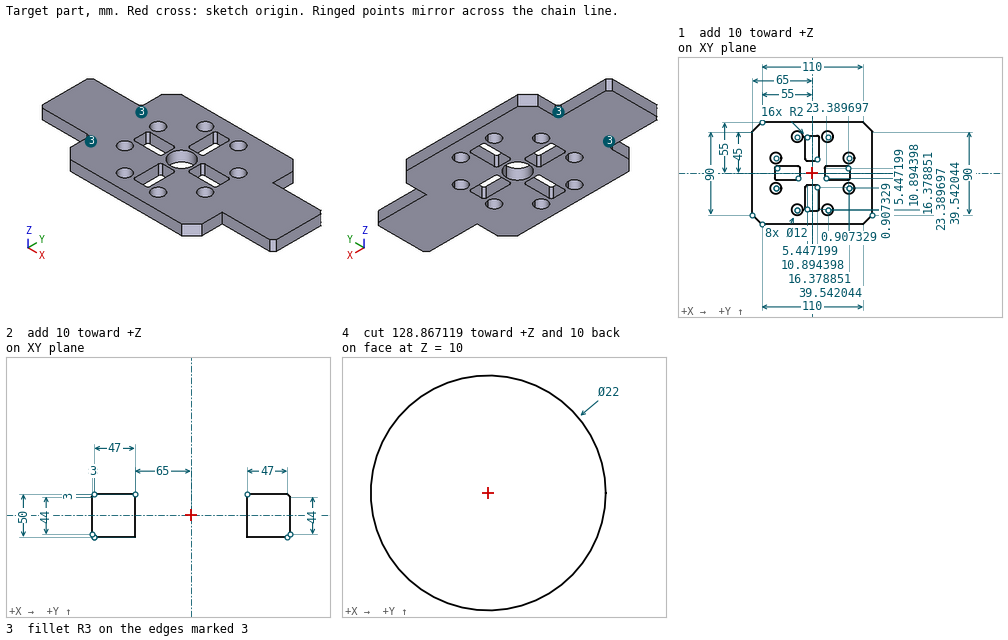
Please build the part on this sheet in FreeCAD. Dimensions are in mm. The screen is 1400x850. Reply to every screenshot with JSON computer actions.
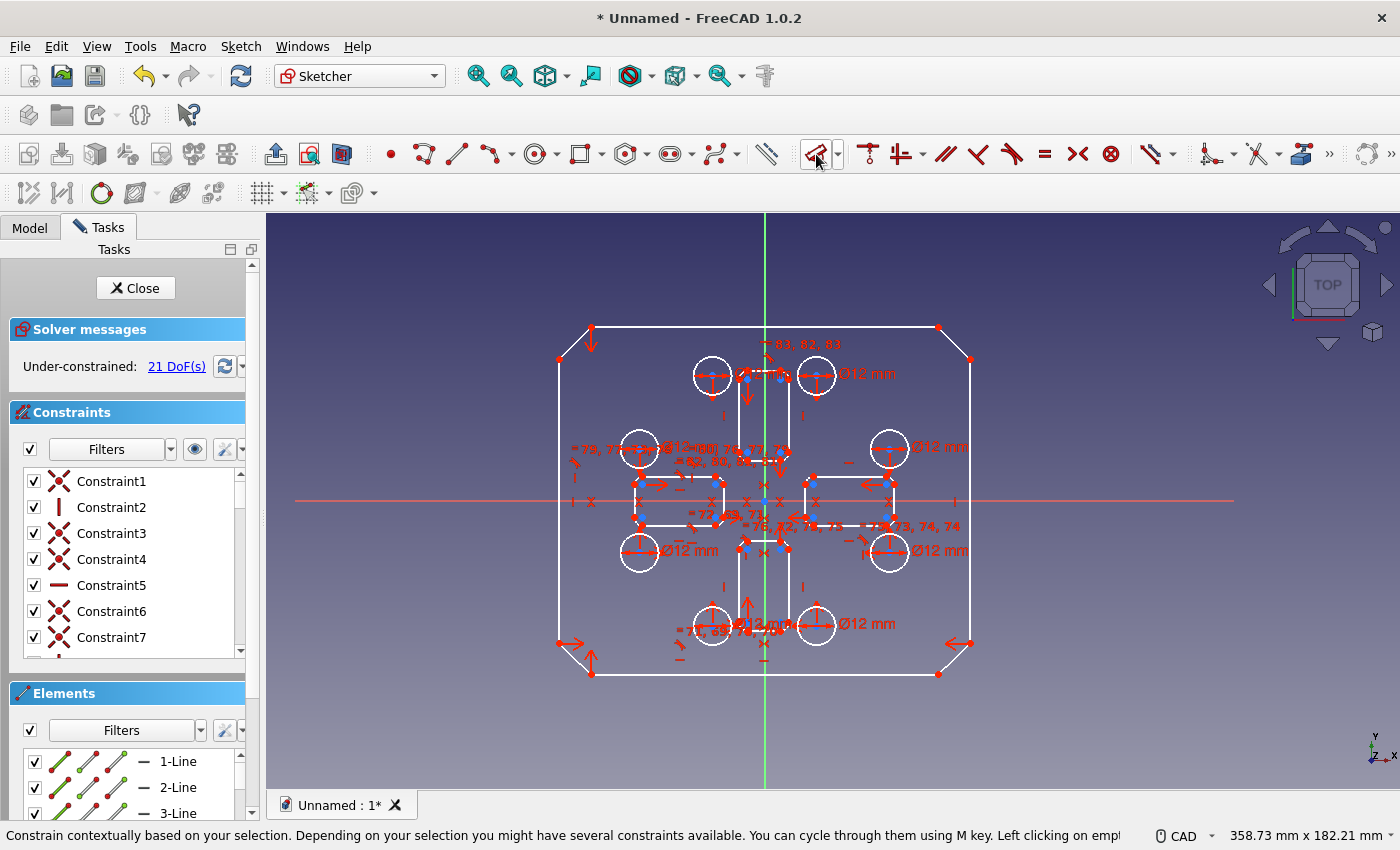
{"action": "scroll", "coordinate": [786, 544], "scroll_direction": "up", "scroll_amount": 10}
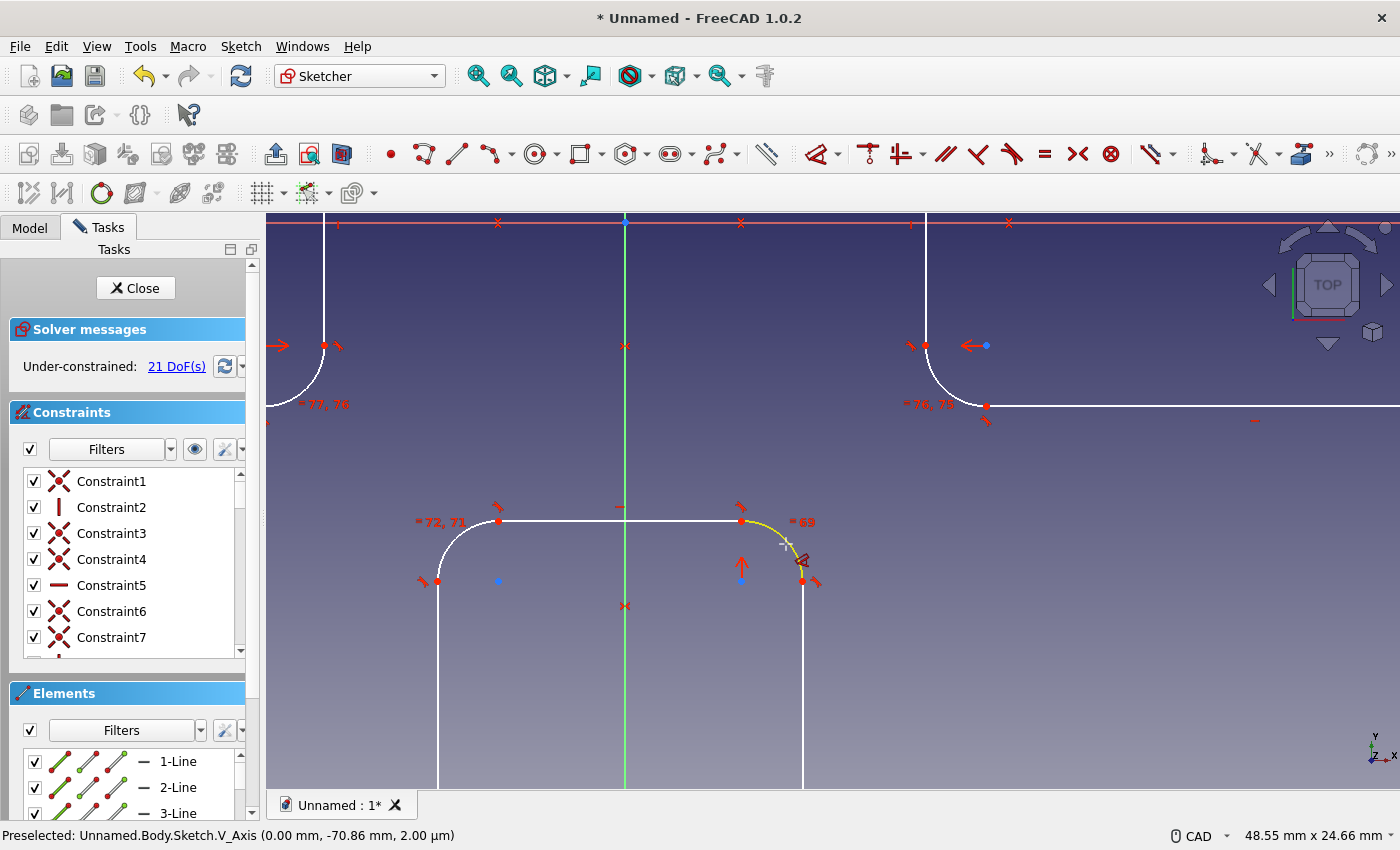
{"action": "left_click", "coordinate": [785, 539]}
{"action": "left_click", "coordinate": [808, 516]}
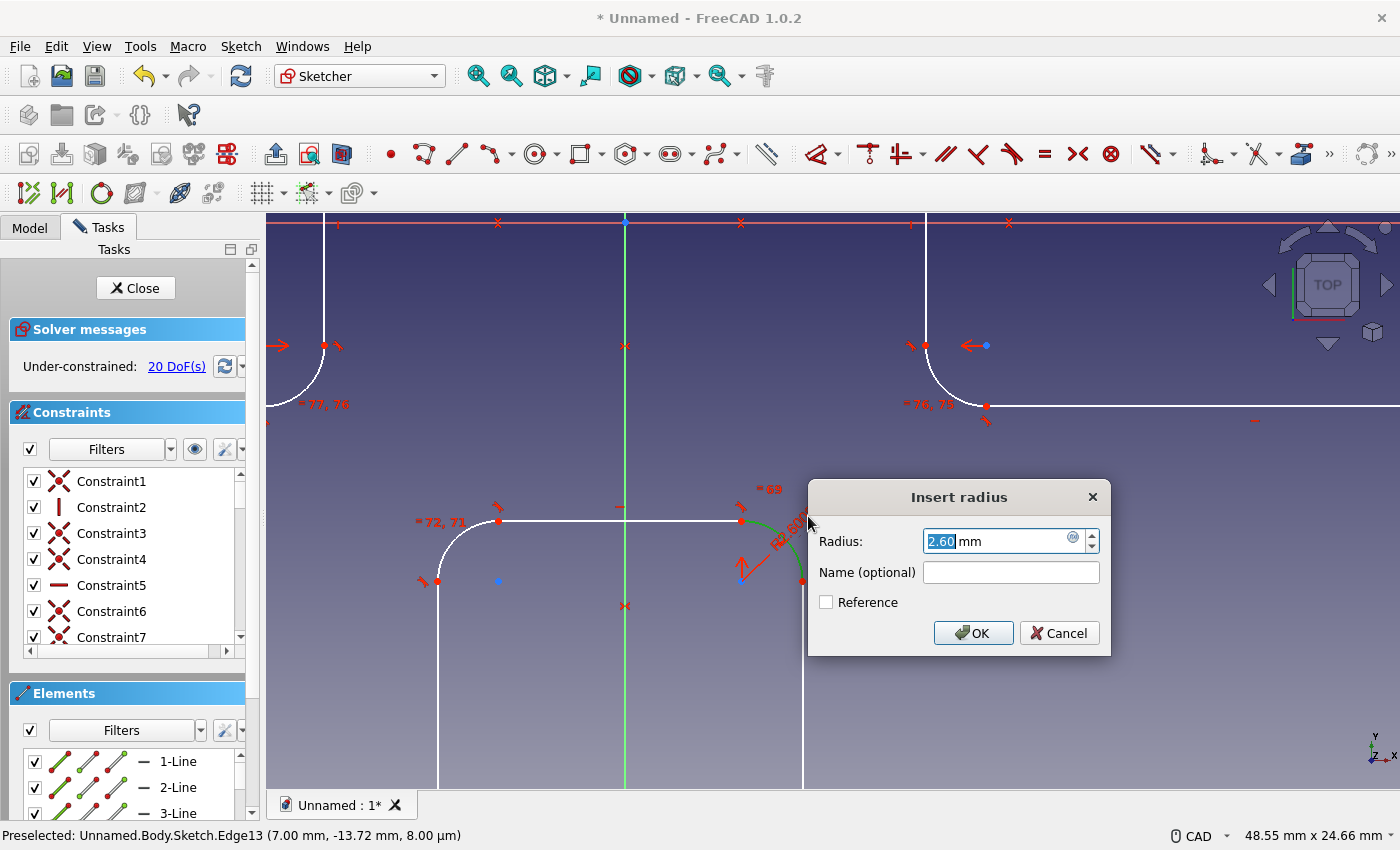
{"action": "type", "text": "2"}
{"action": "key", "text": "Return"}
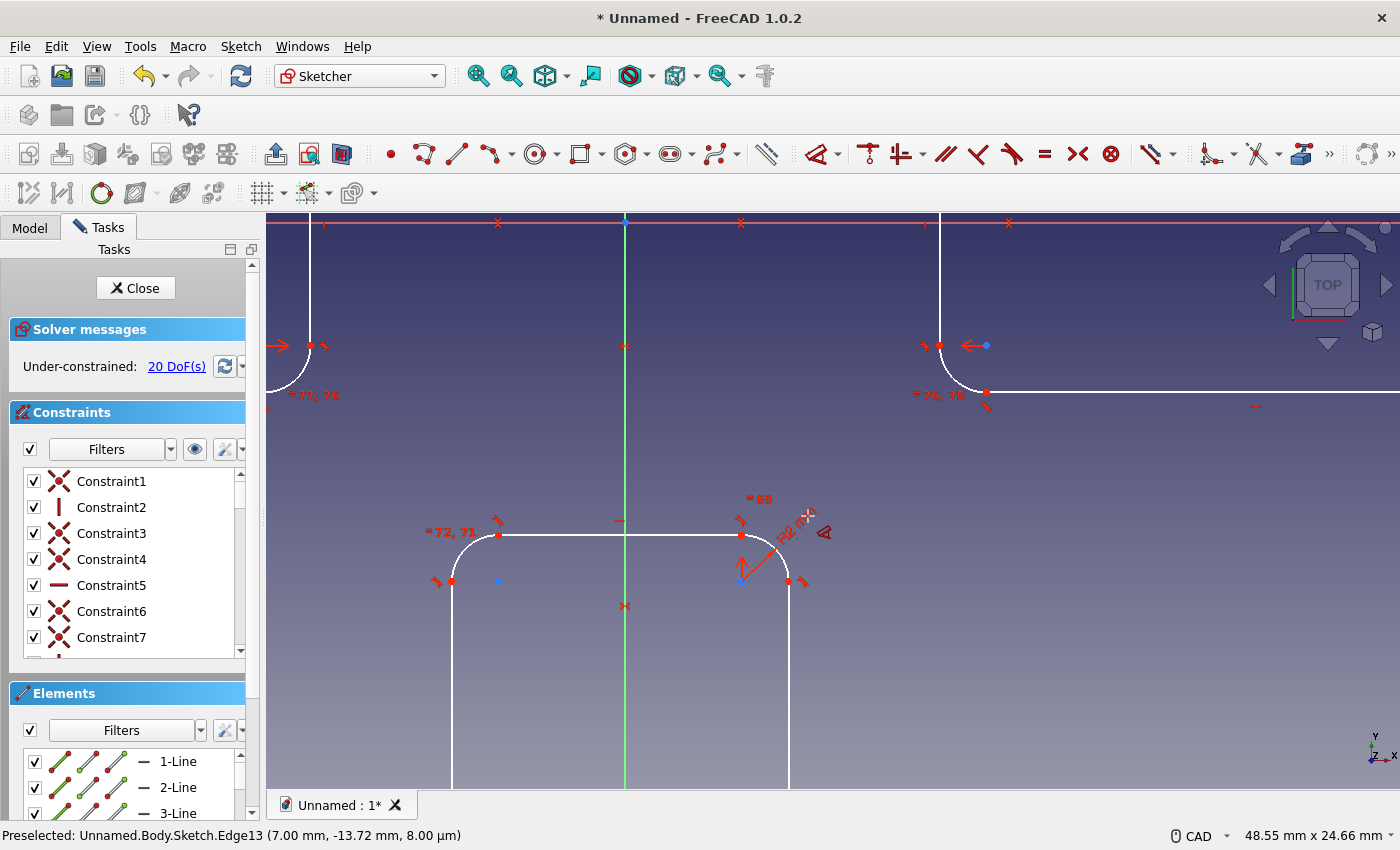
{"action": "scroll", "coordinate": [786, 545], "scroll_direction": "down", "scroll_amount": 10}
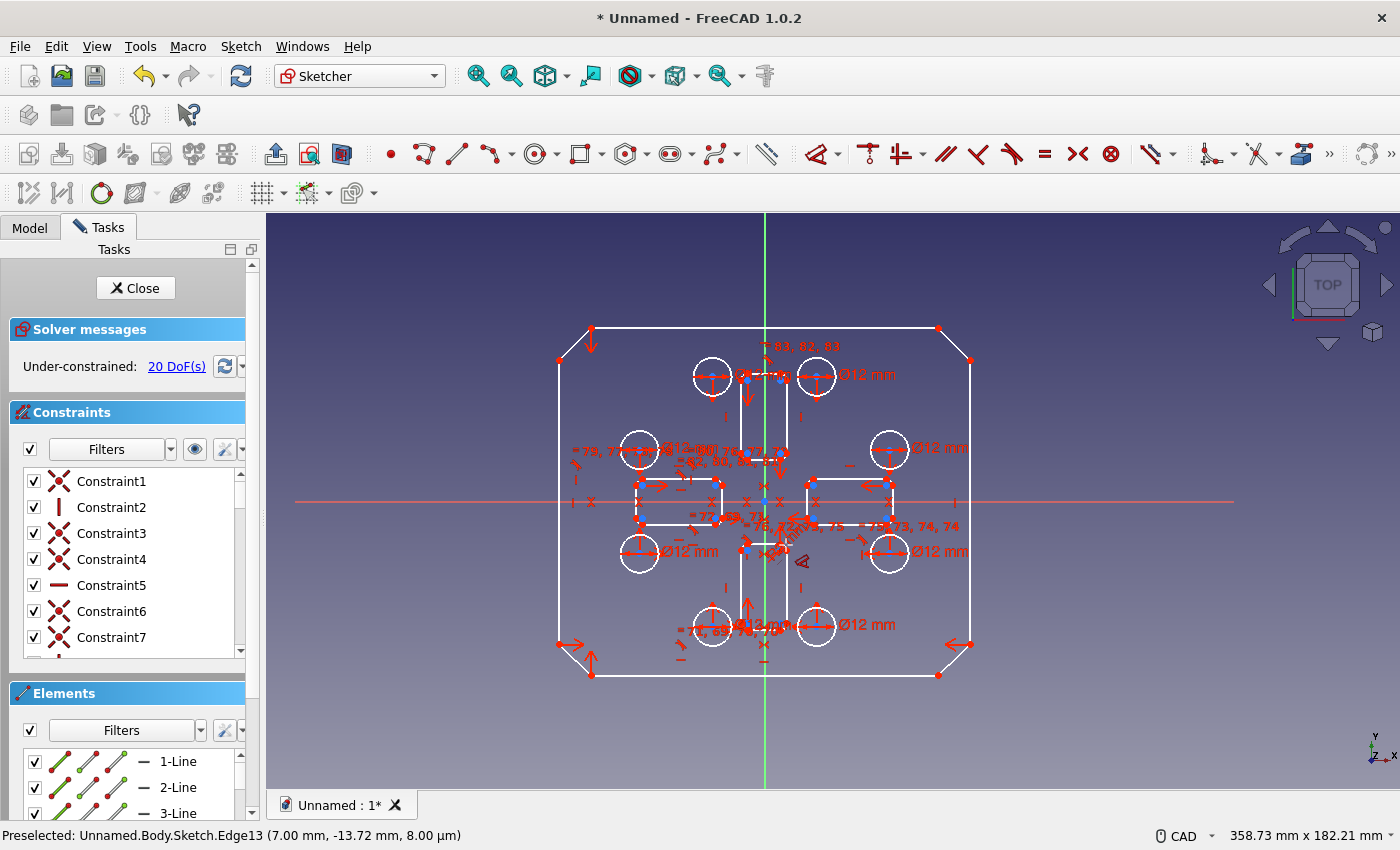
{"action": "left_click", "coordinate": [559, 446]}
{"action": "left_click", "coordinate": [525, 437]}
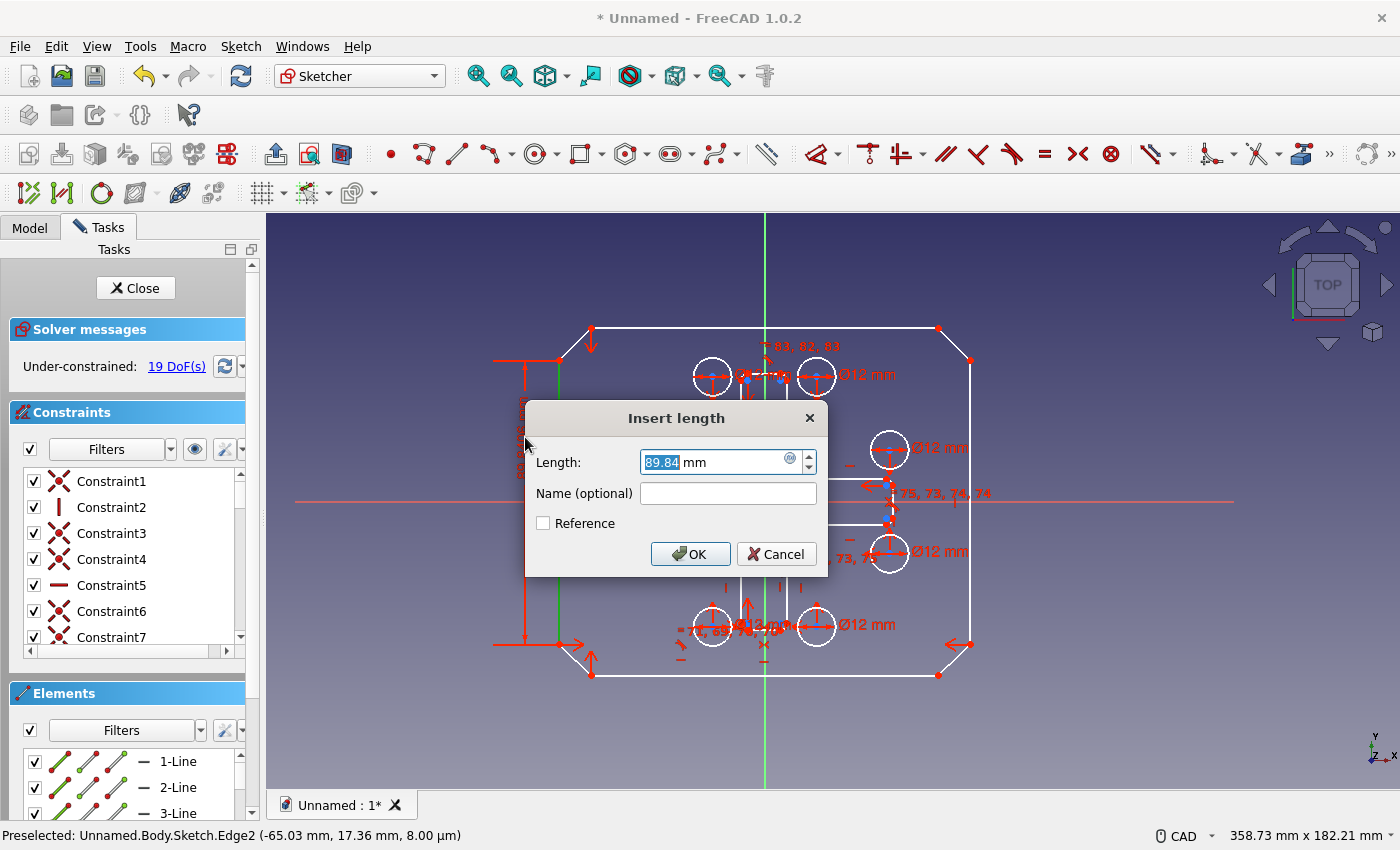
{"action": "type", "text": "90"}
{"action": "key", "text": "Return"}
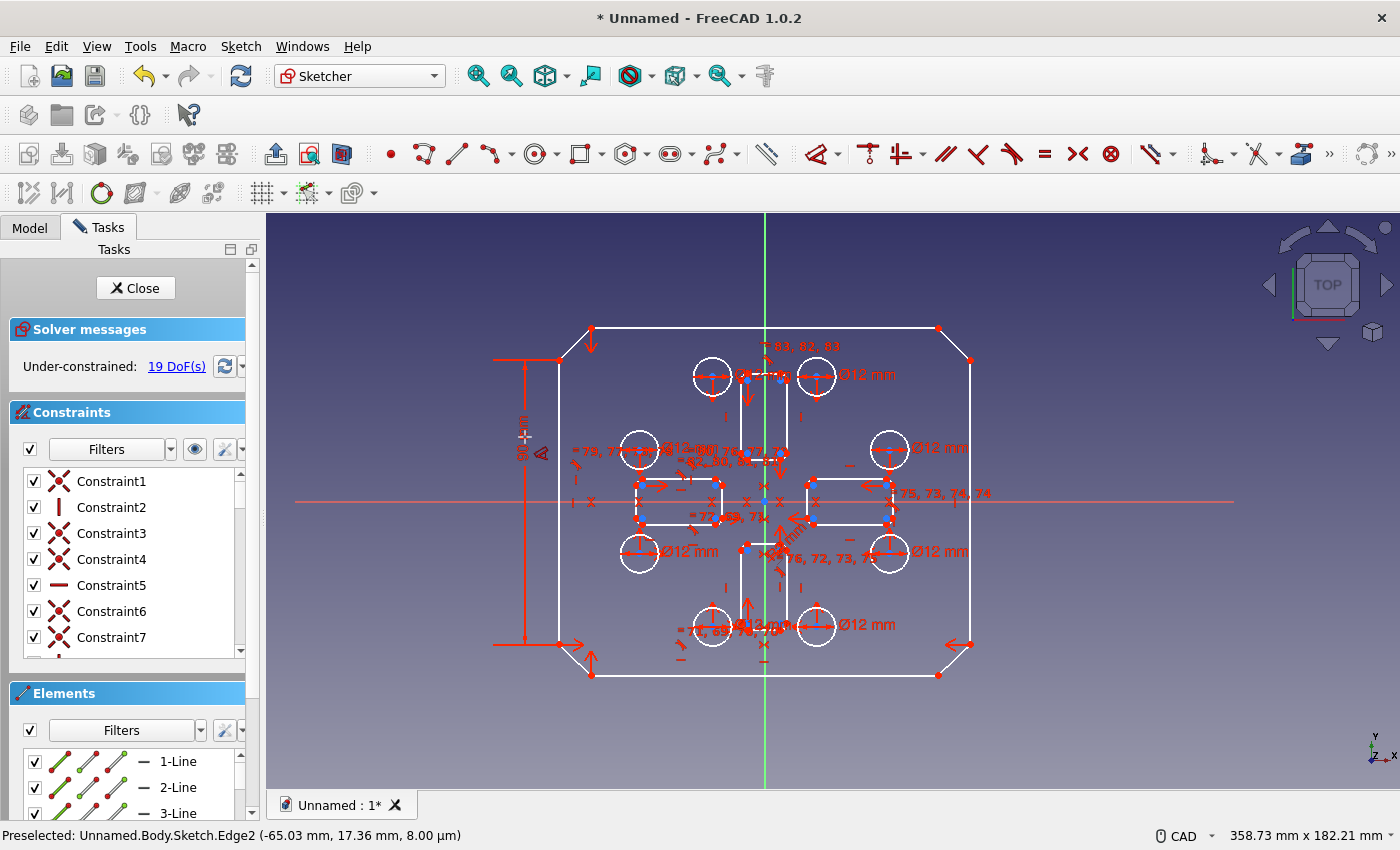
{"action": "left_click", "coordinate": [970, 560]}
{"action": "left_click", "coordinate": [1004, 437]}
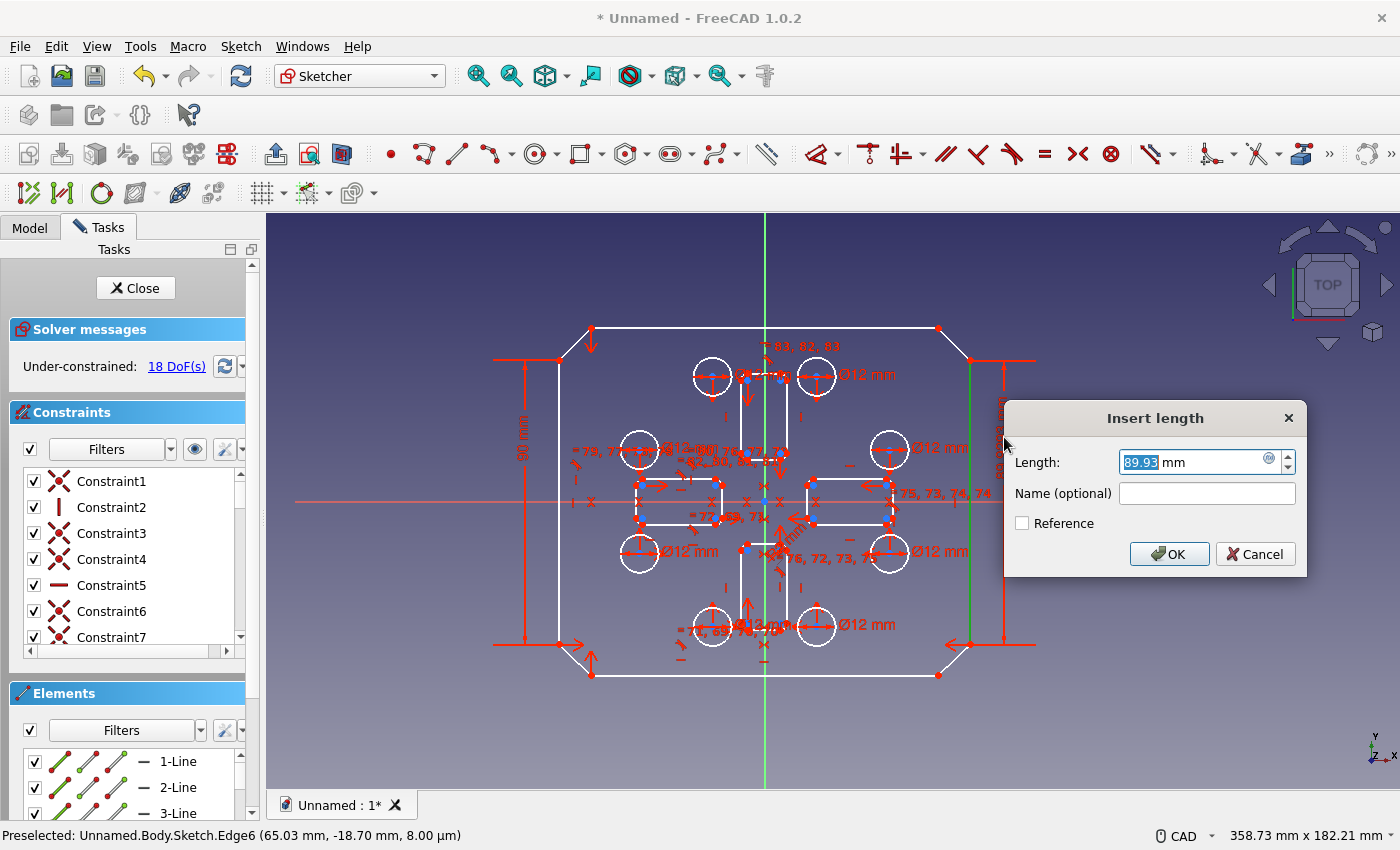
{"action": "type", "text": "90"}
{"action": "key", "text": "Return"}